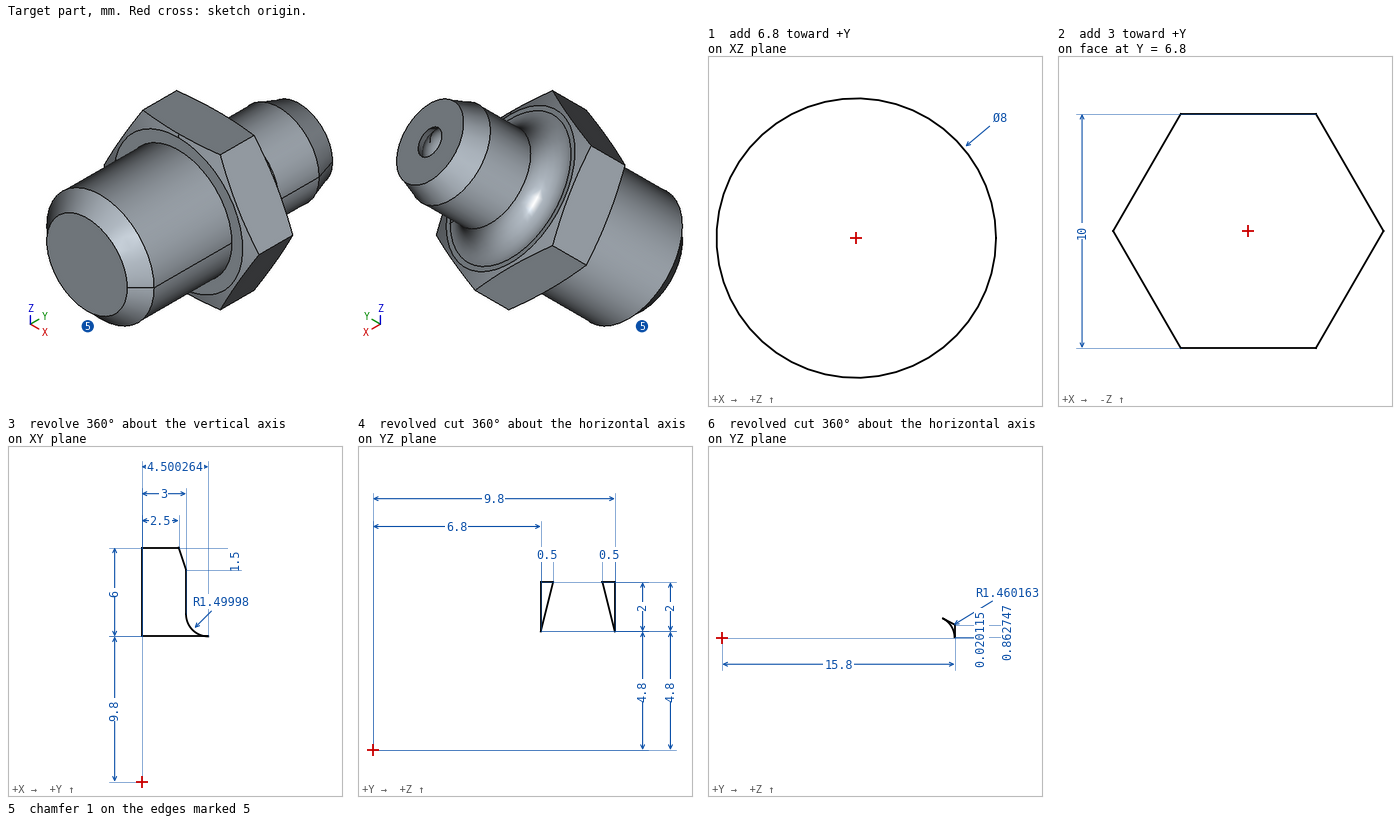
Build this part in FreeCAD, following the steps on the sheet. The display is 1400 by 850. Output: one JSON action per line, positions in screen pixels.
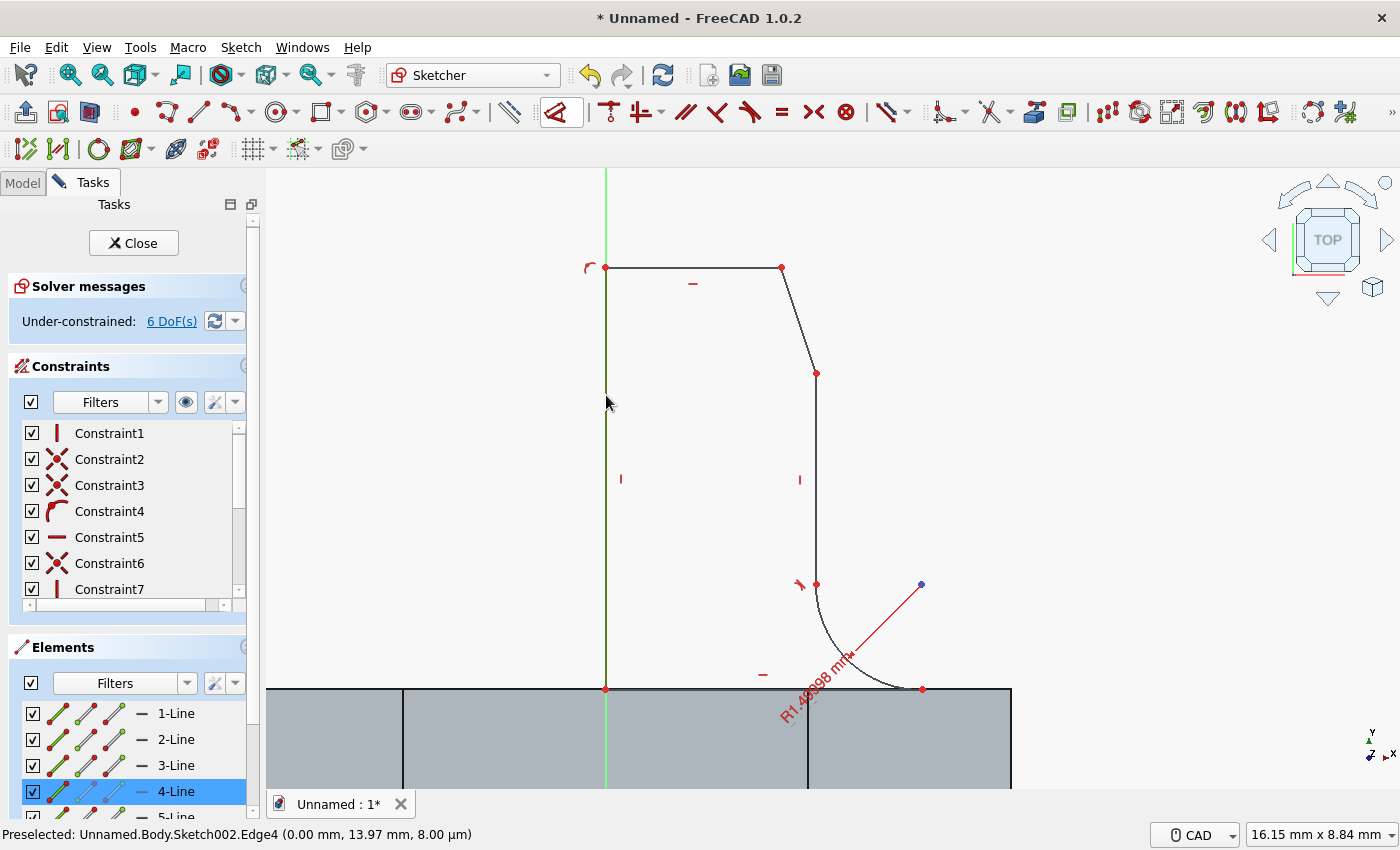
{"action": "key", "text": "i"}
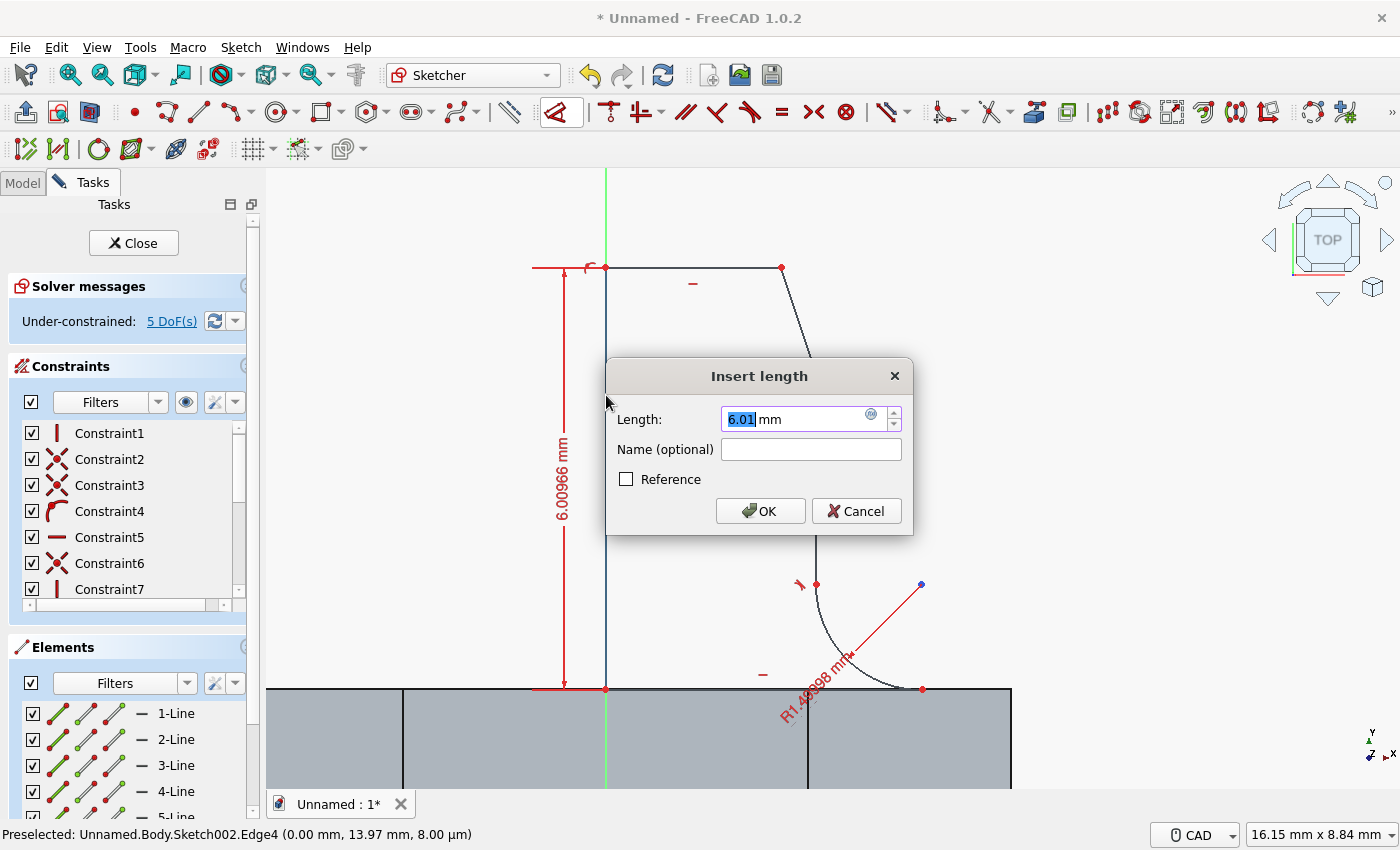
{"action": "type", "text": "6"}
{"action": "key", "text": "Return"}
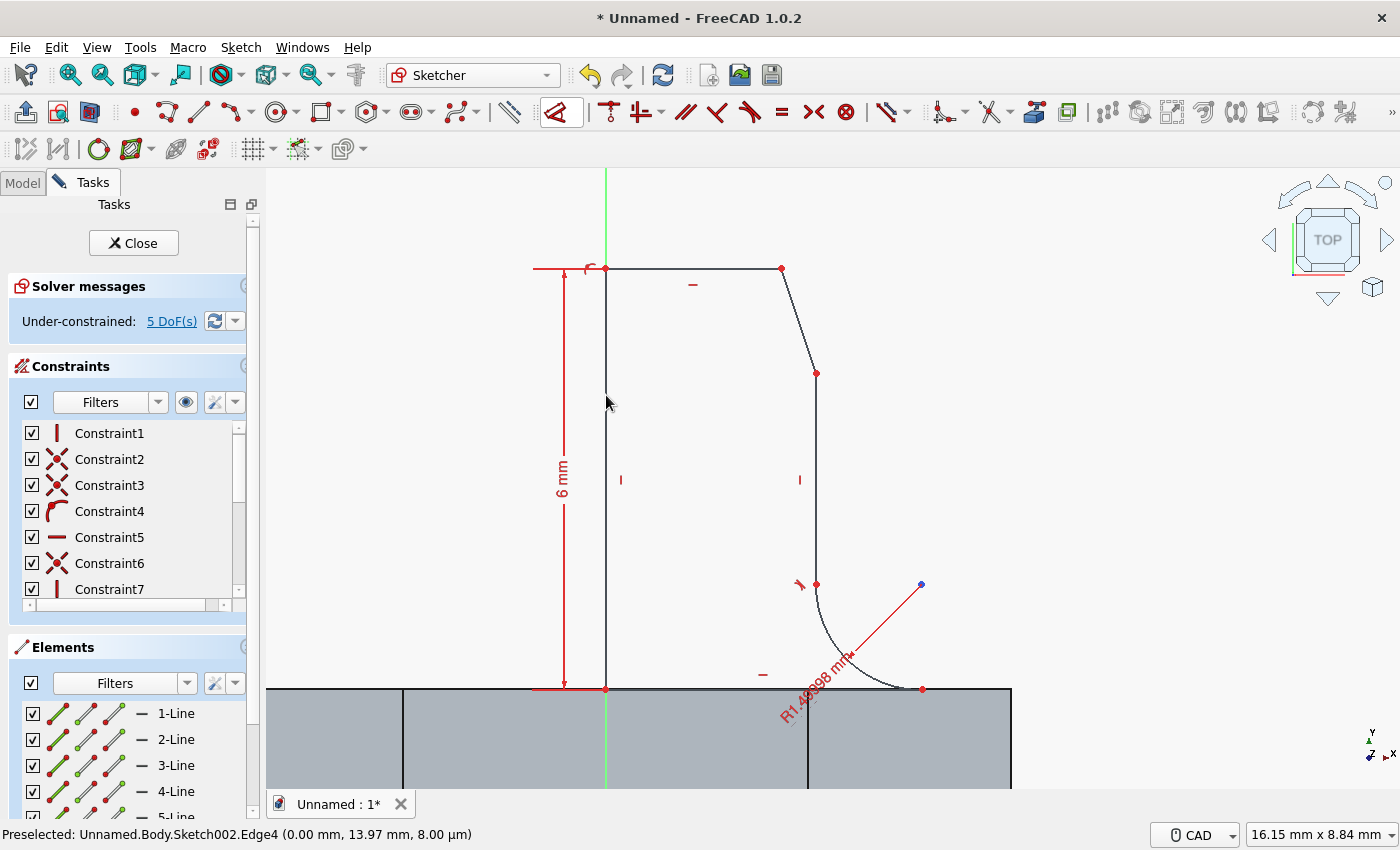
{"action": "left_click", "coordinate": [816, 585]}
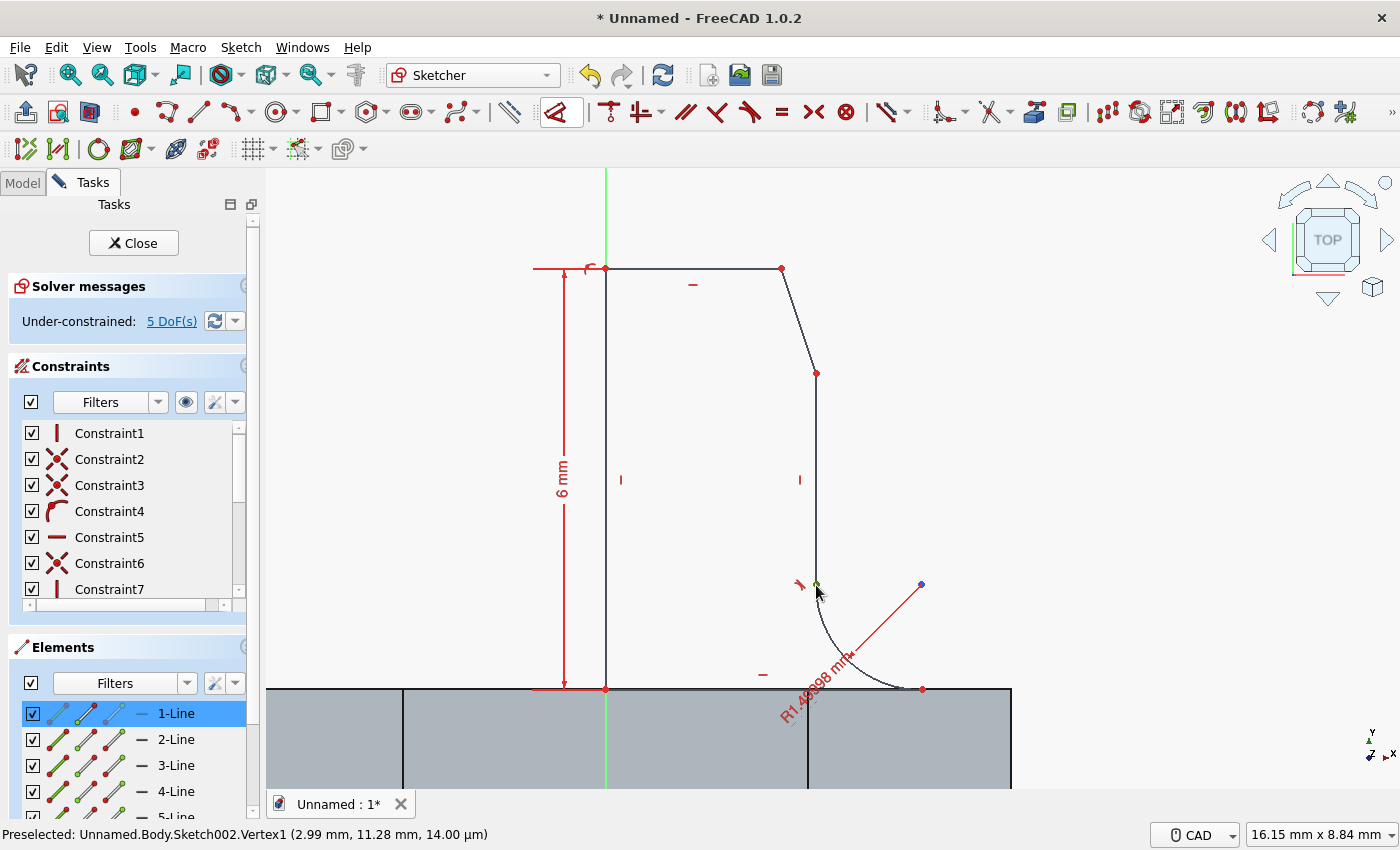
{"action": "key", "text": "l"}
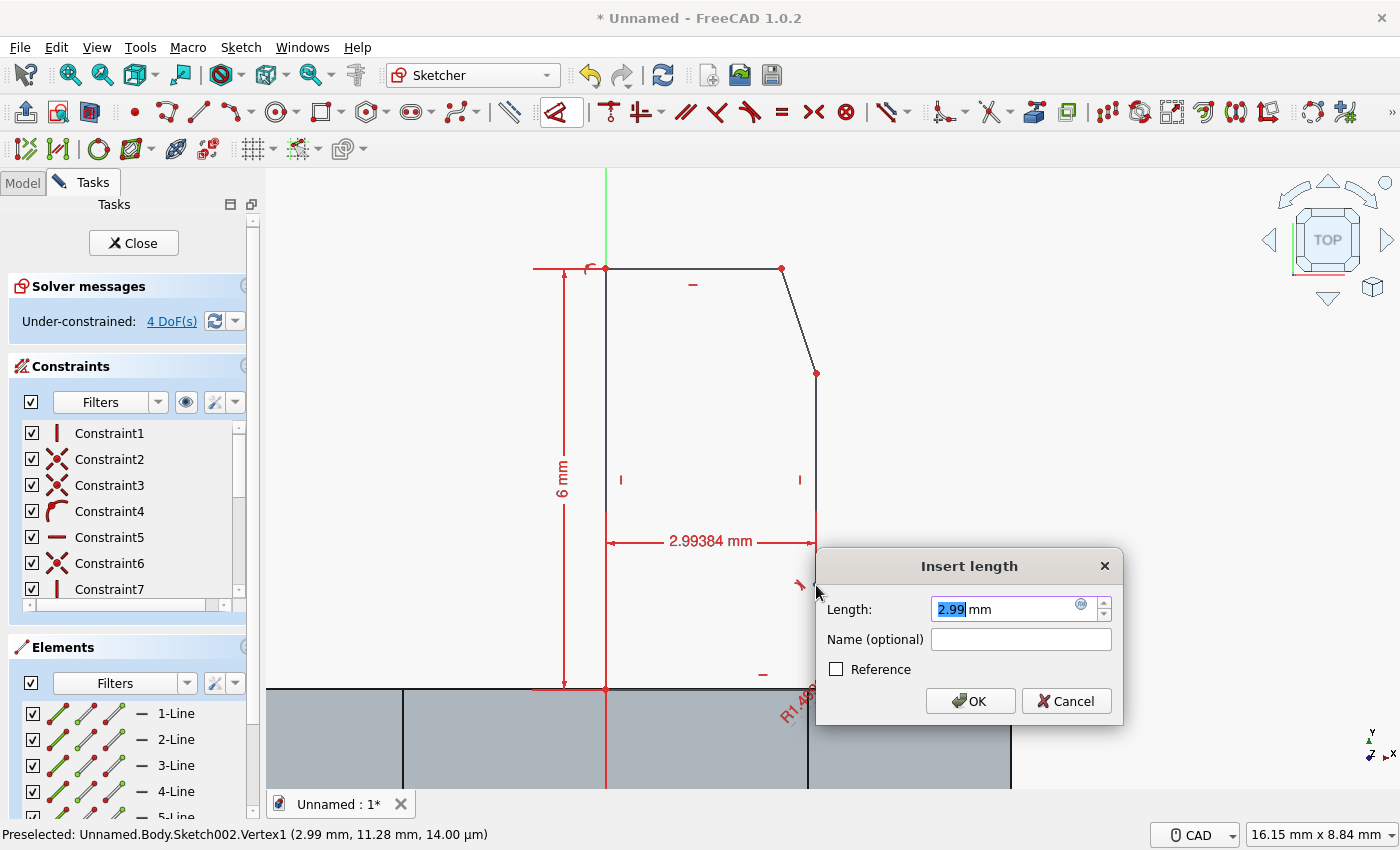
{"action": "type", "text": "3"}
{"action": "key", "text": "Return"}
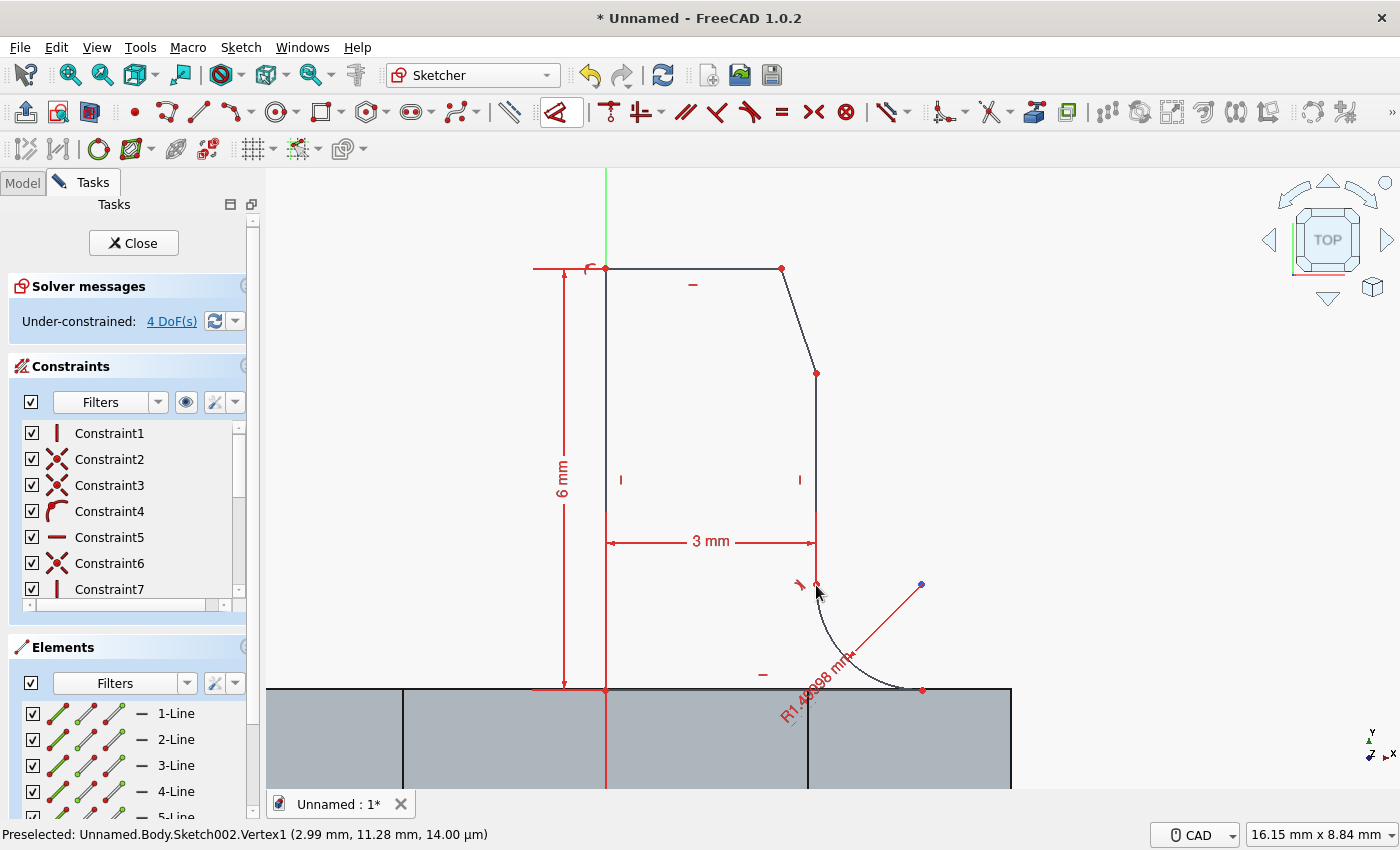
{"action": "left_click", "coordinate": [728, 269]}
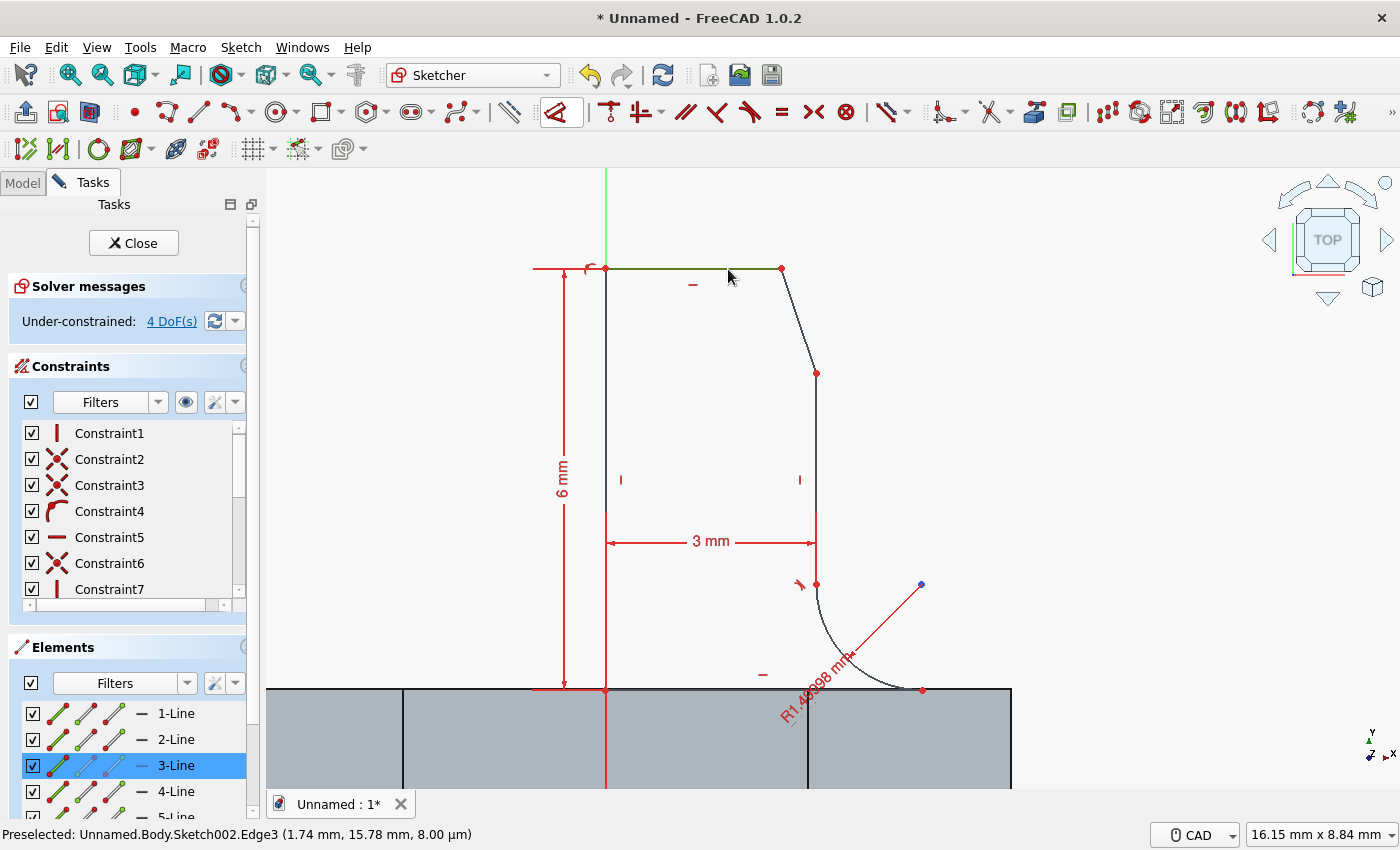
{"action": "key", "text": "l"}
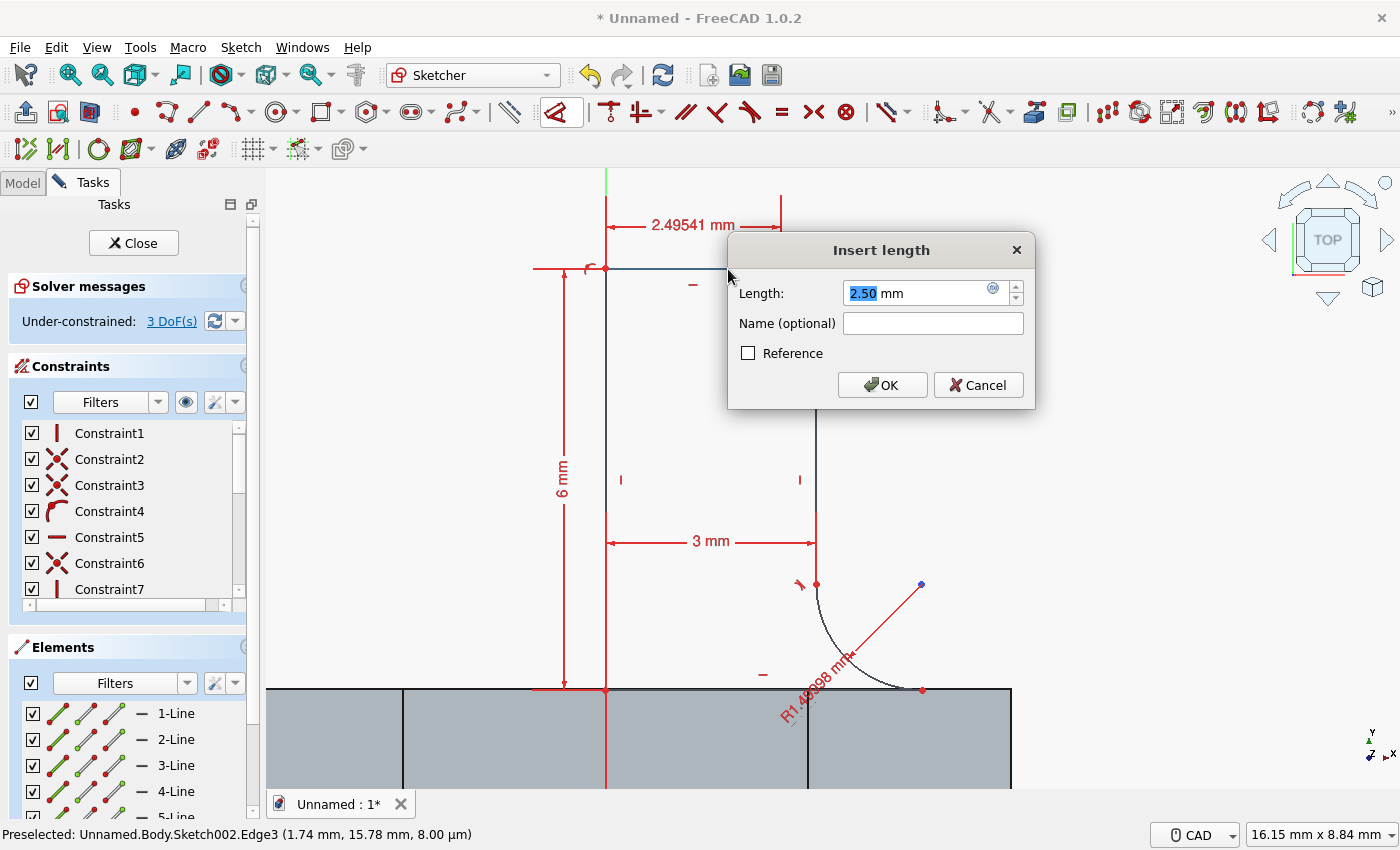
{"action": "type", "text": "2.5"}
{"action": "key", "text": "Return"}